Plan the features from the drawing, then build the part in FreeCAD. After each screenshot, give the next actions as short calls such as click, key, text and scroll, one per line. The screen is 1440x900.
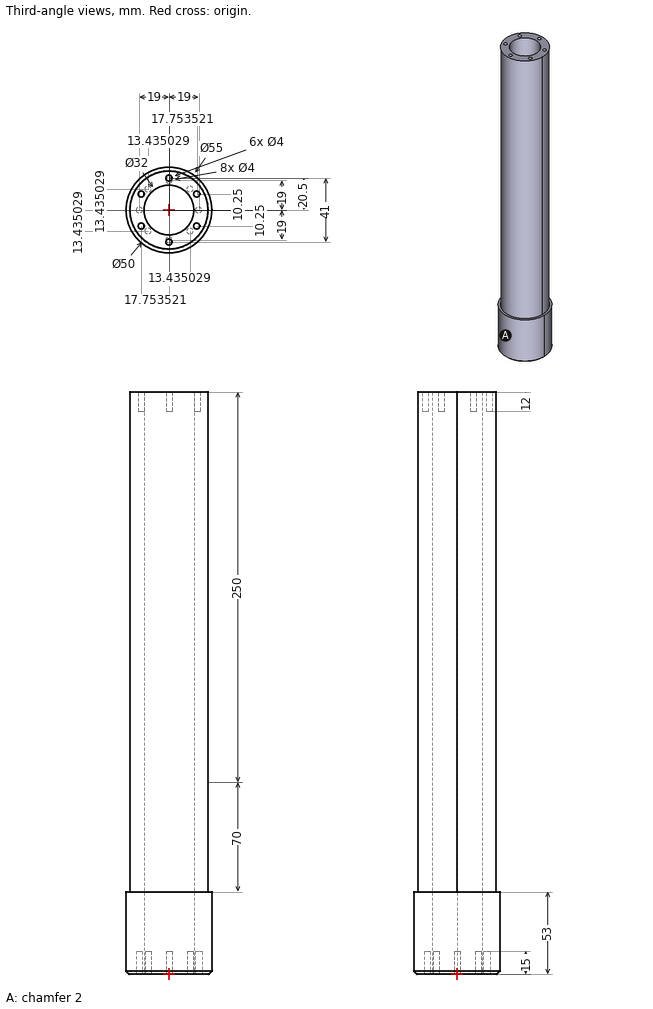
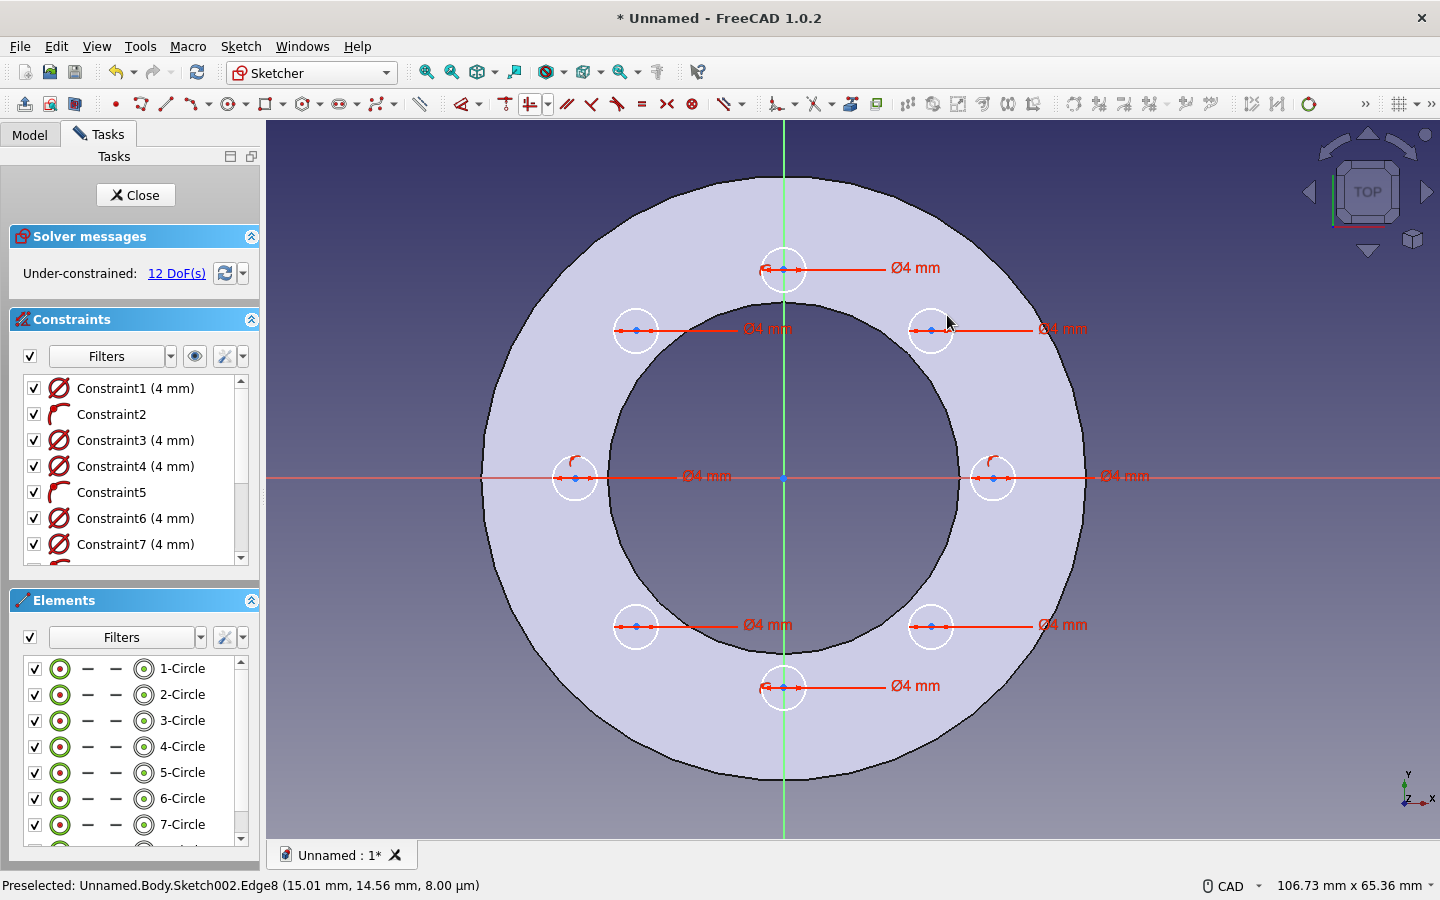
click(636, 331)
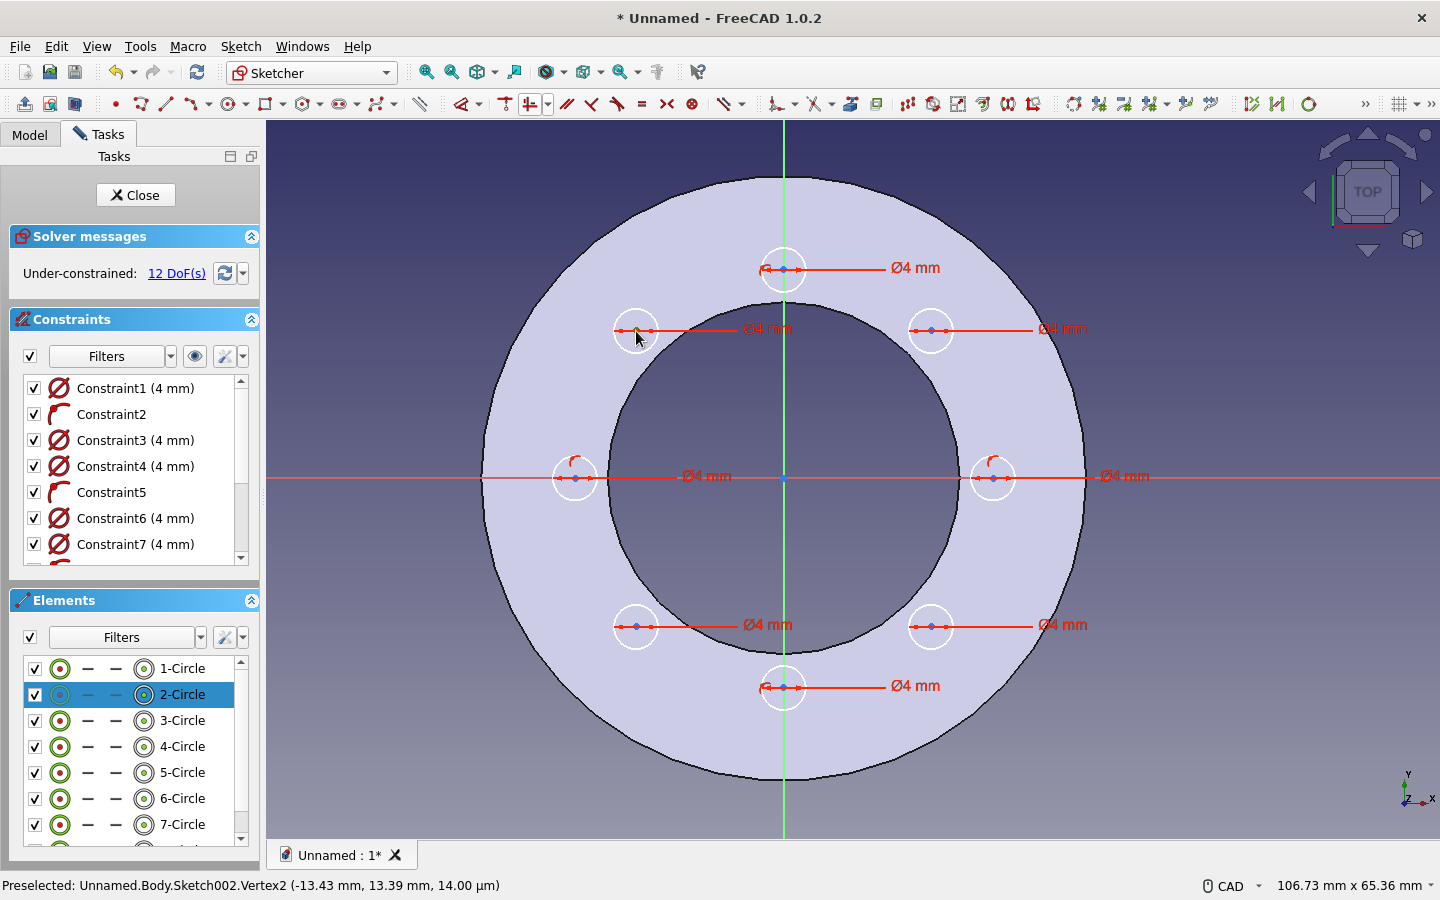
click(636, 627)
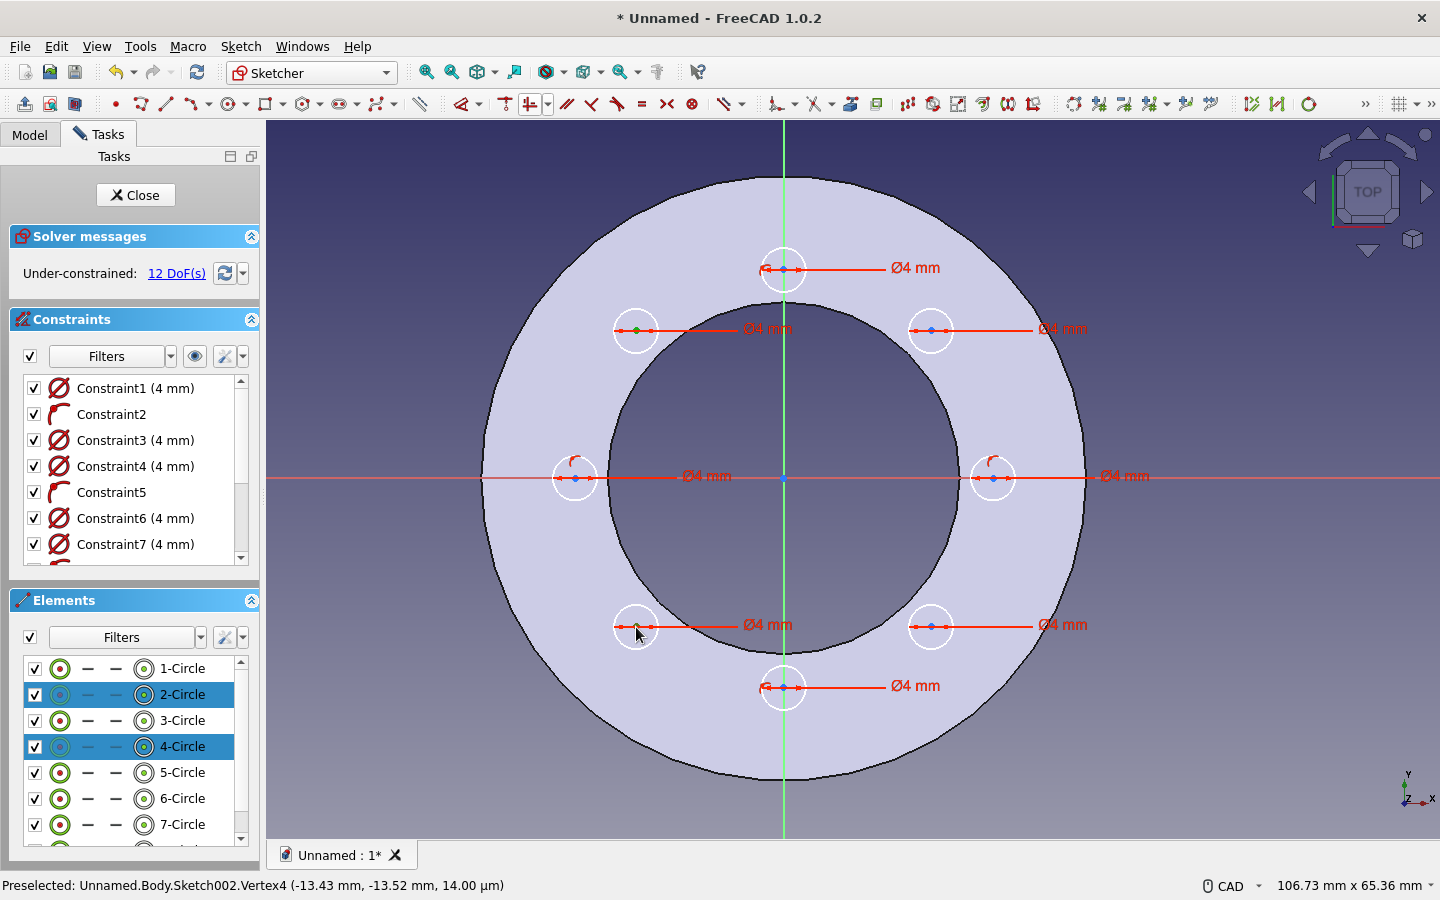
key(v)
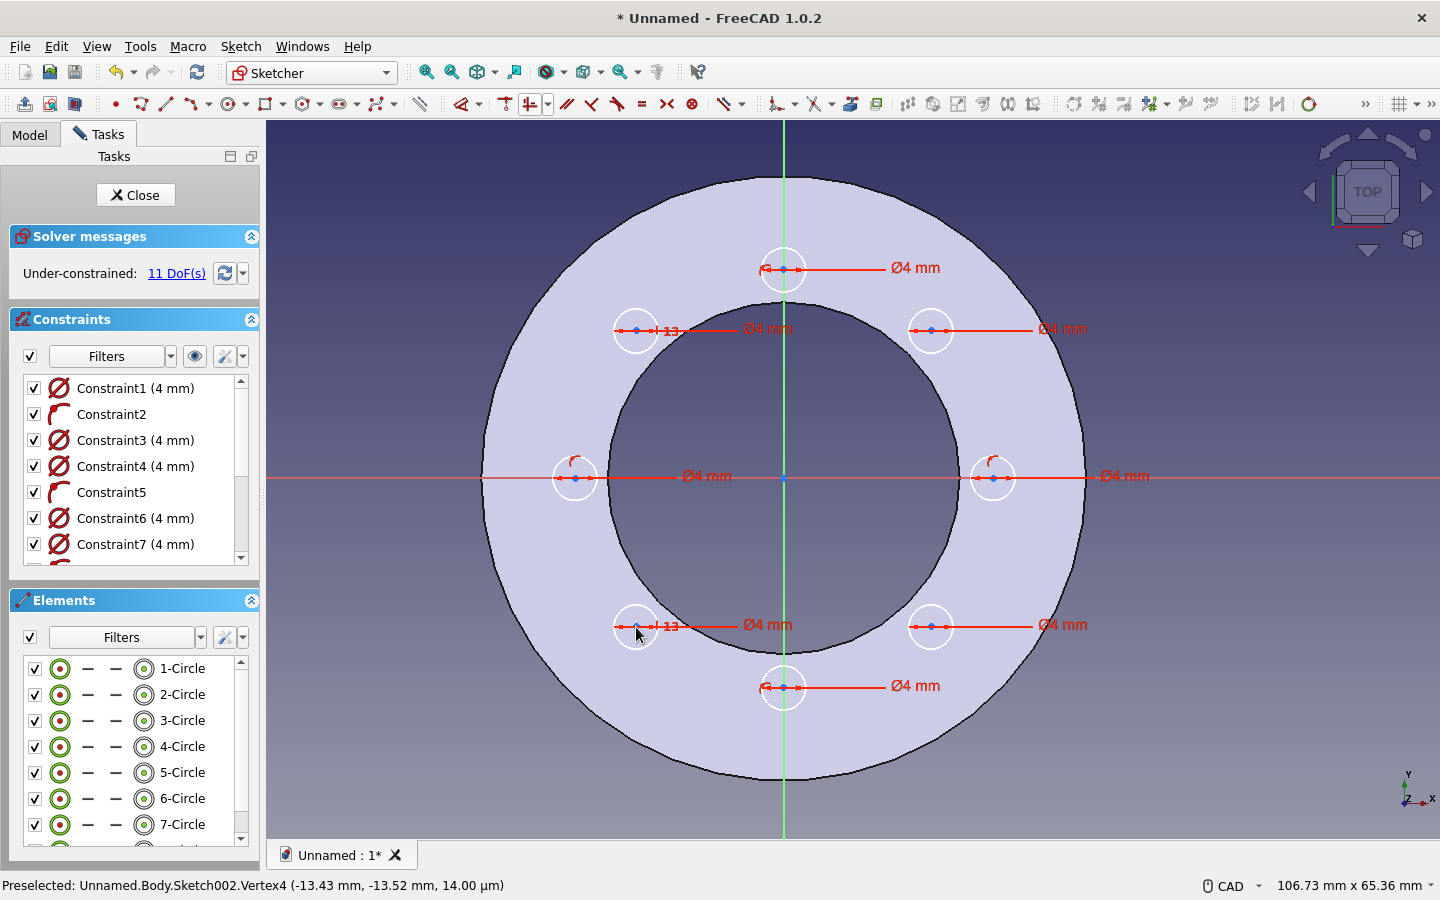
click(636, 627)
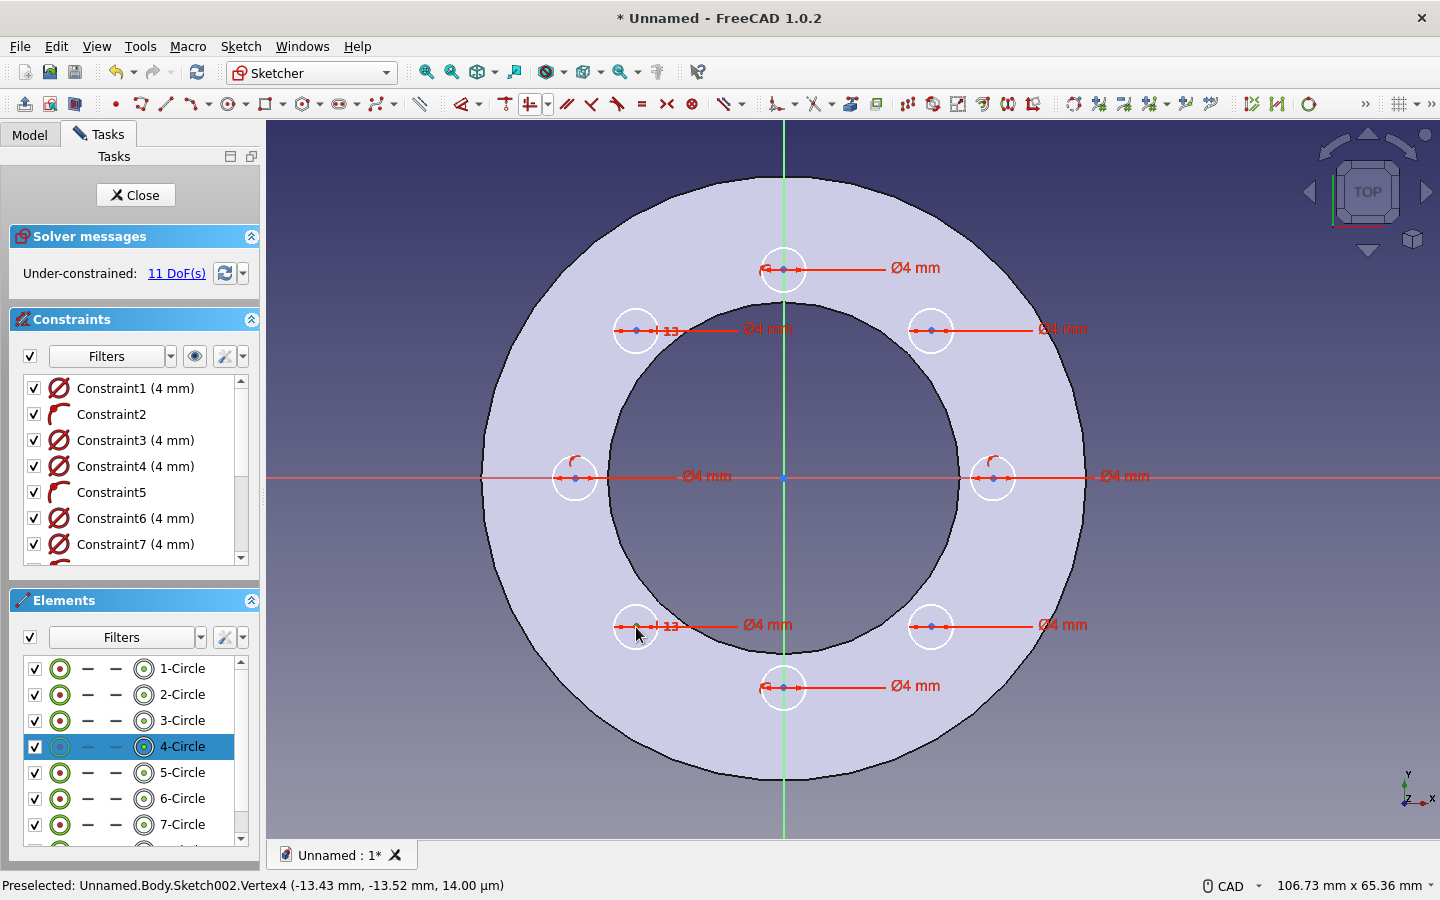
click(931, 627)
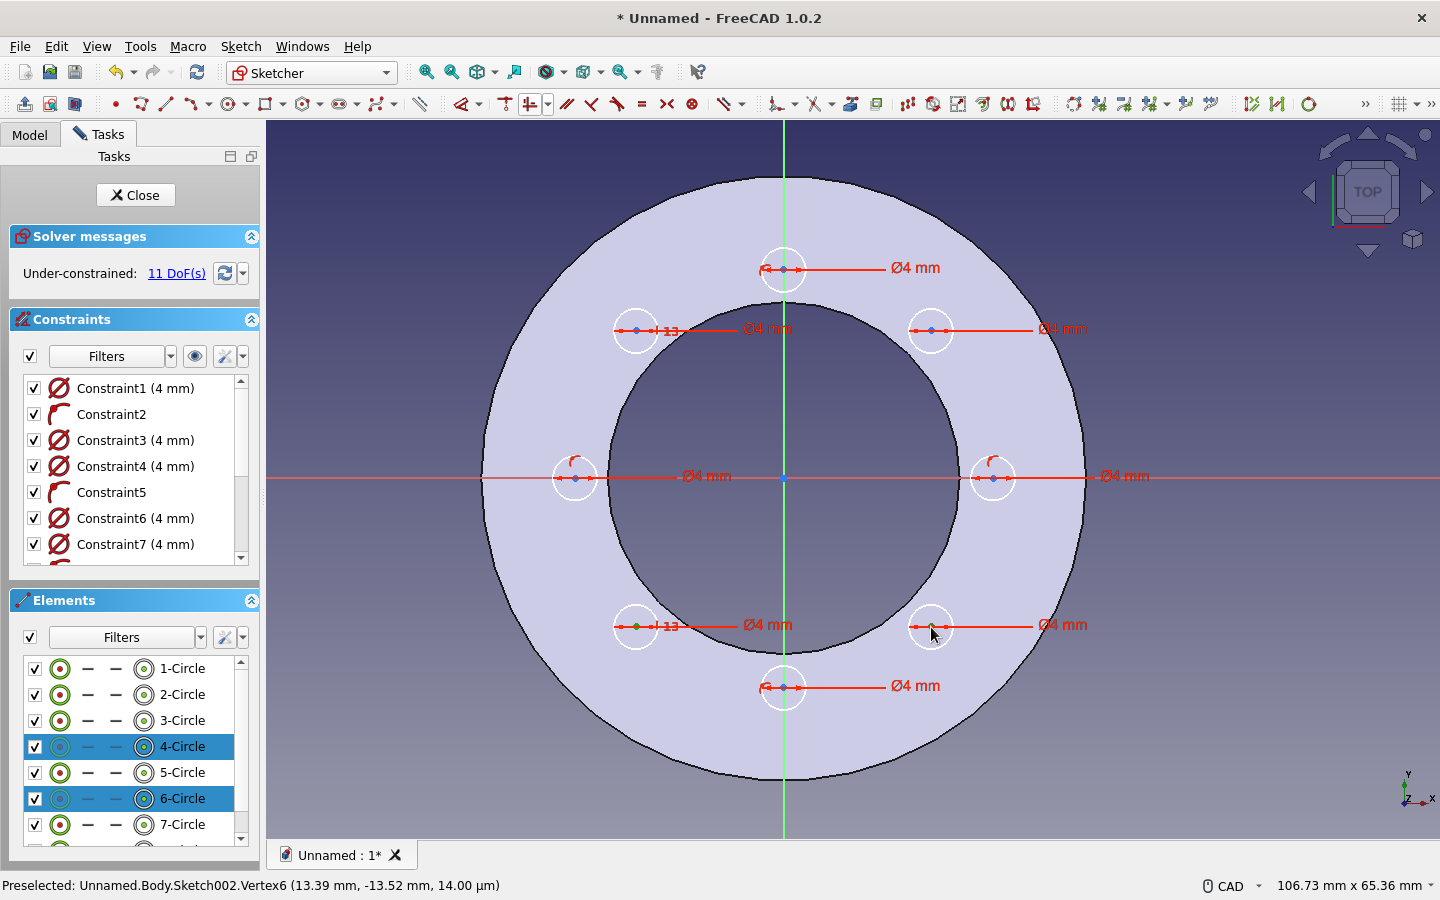
click(548, 104)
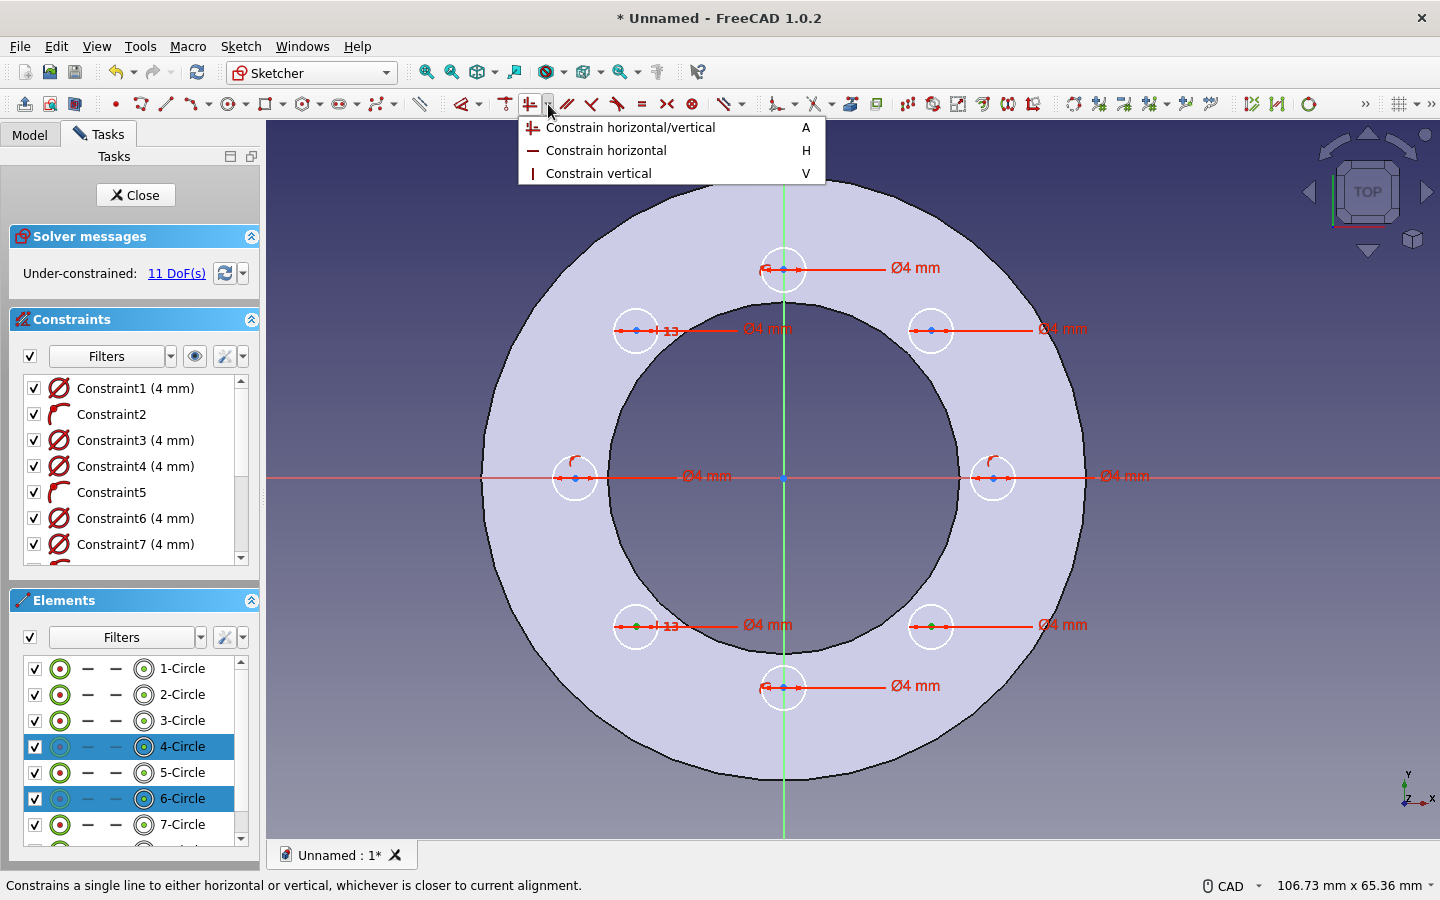
click(672, 150)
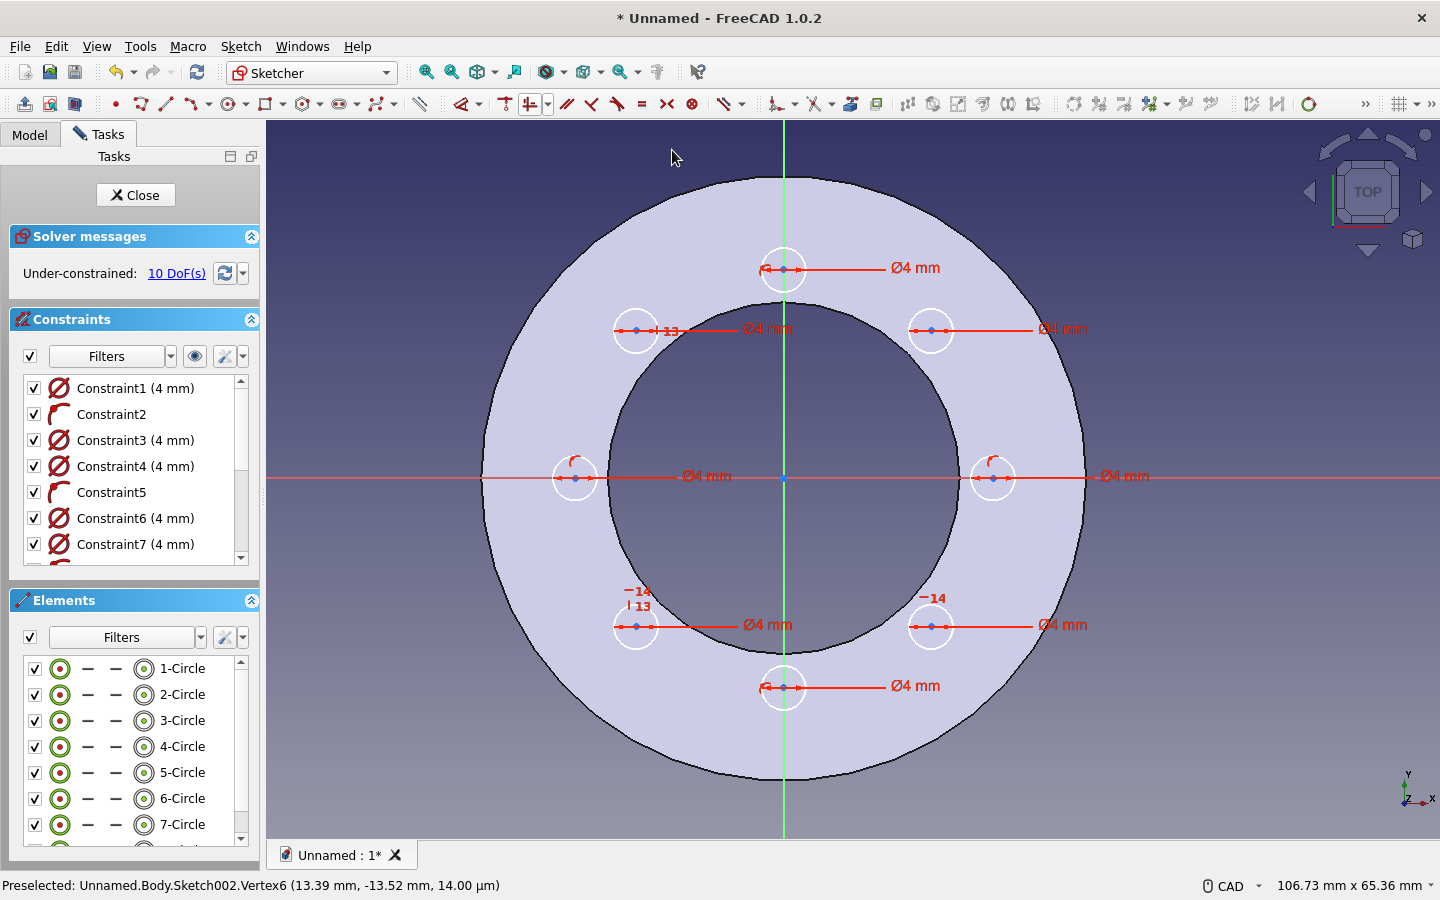
click(931, 627)